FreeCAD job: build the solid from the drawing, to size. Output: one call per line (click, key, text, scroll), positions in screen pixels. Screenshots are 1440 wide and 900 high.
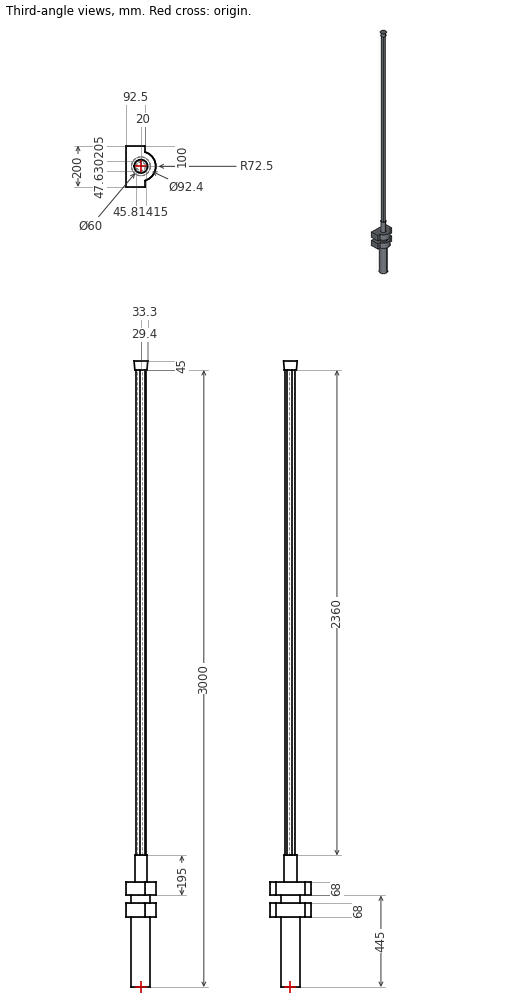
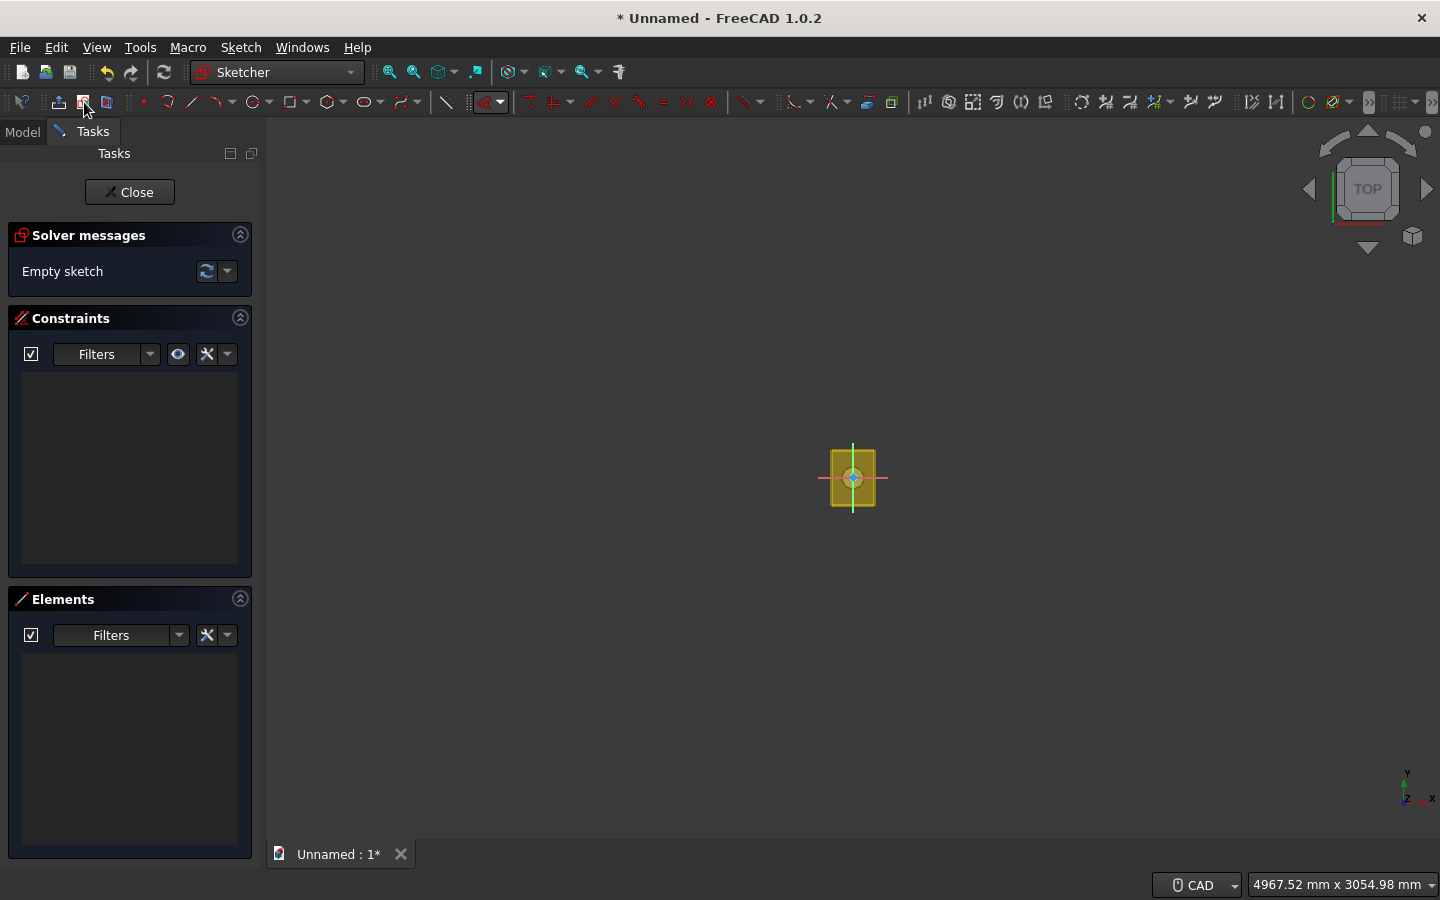
scroll(862, 478, up, 11)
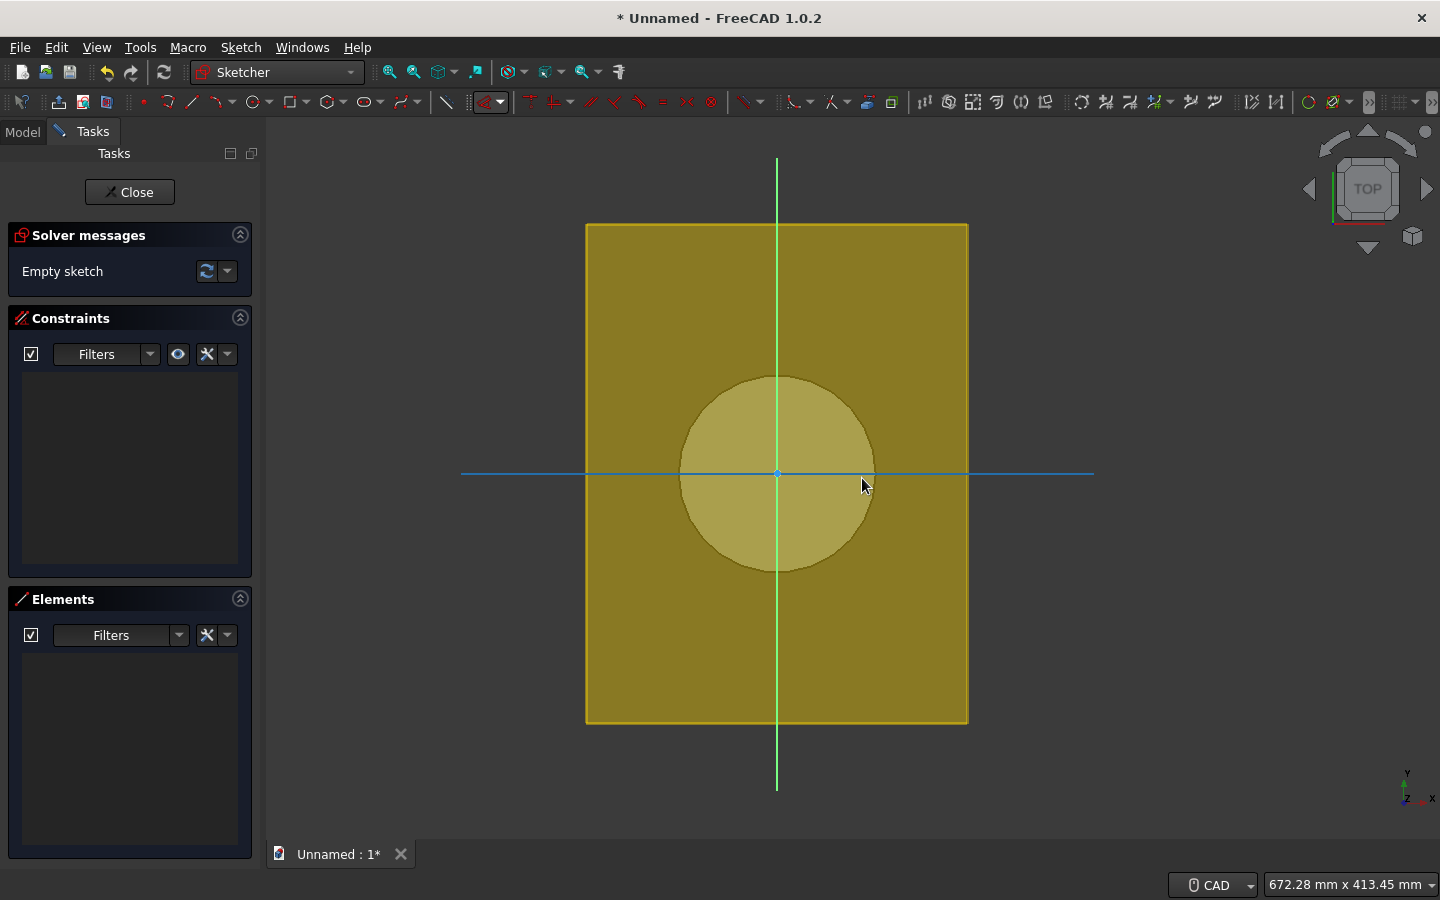
key(g)
key(m)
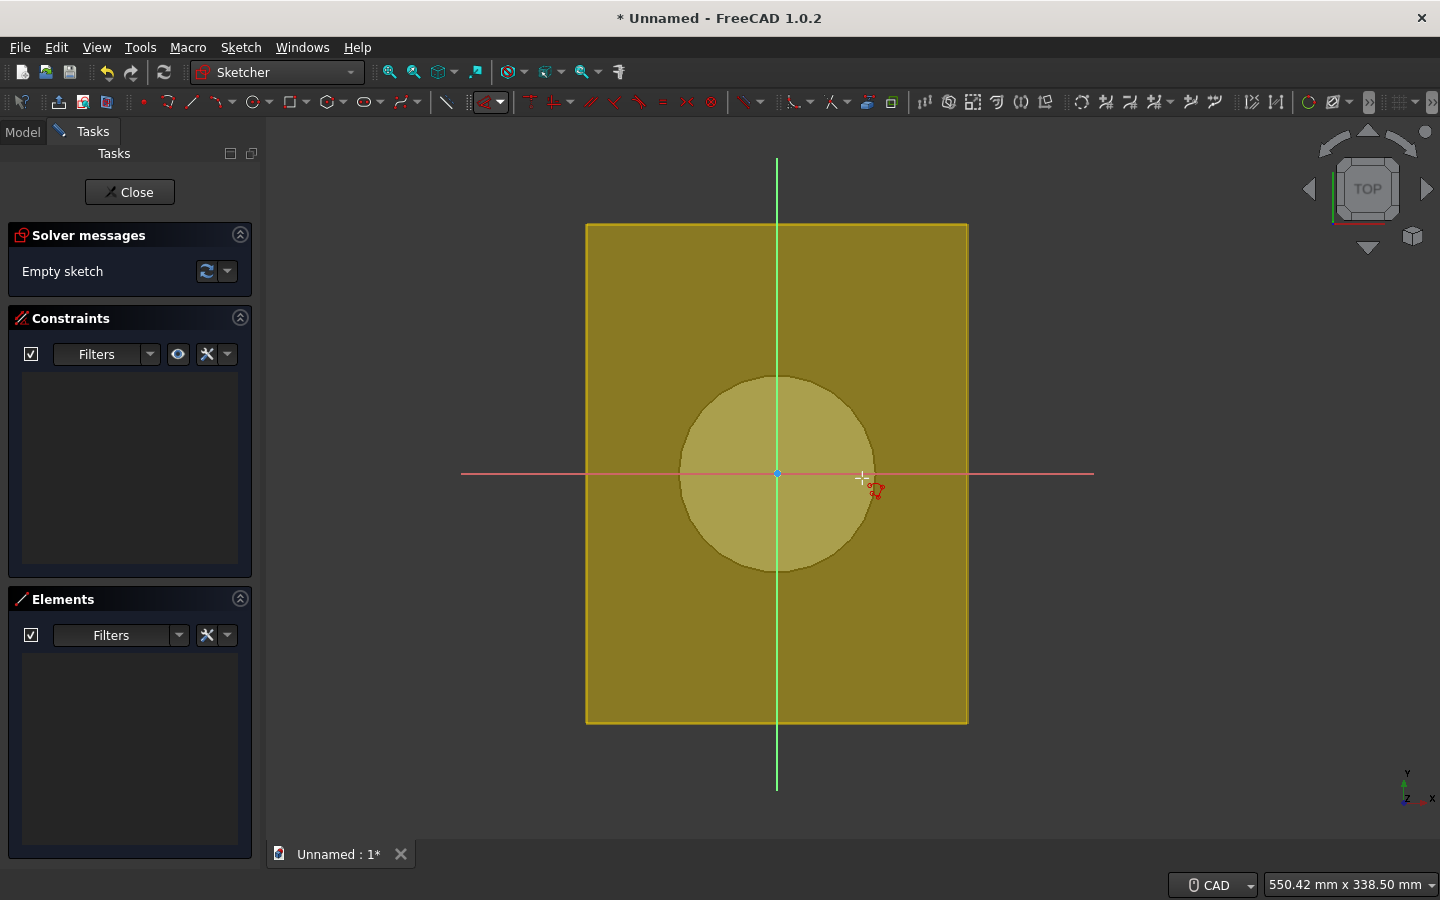
click(820, 325)
click(820, 261)
click(623, 261)
click(623, 687)
click(820, 687)
click(820, 623)
right_click(820, 623)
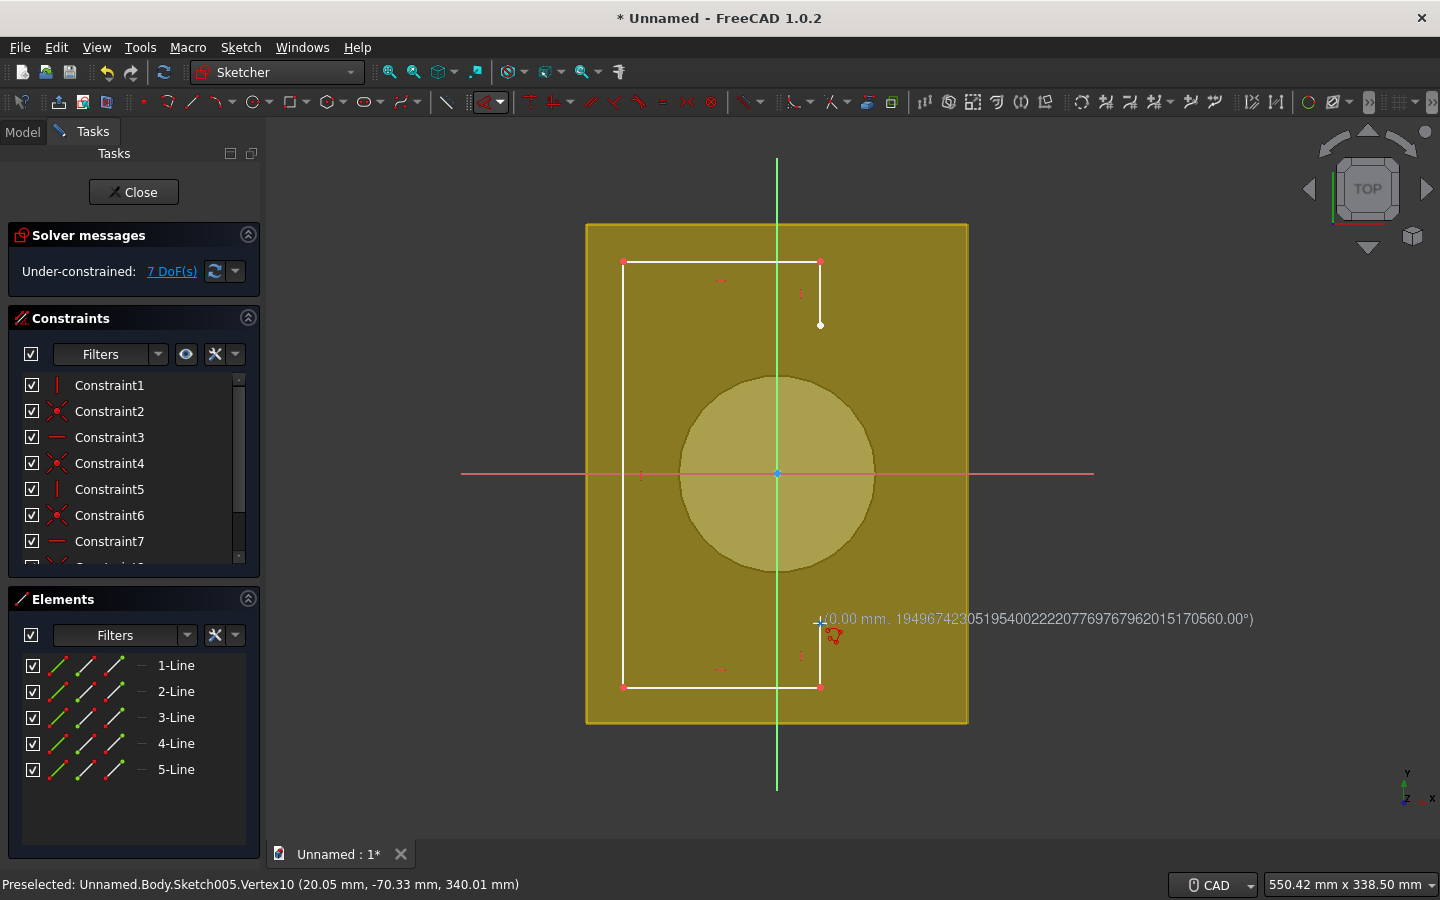
key(g)
key(3)
key(a)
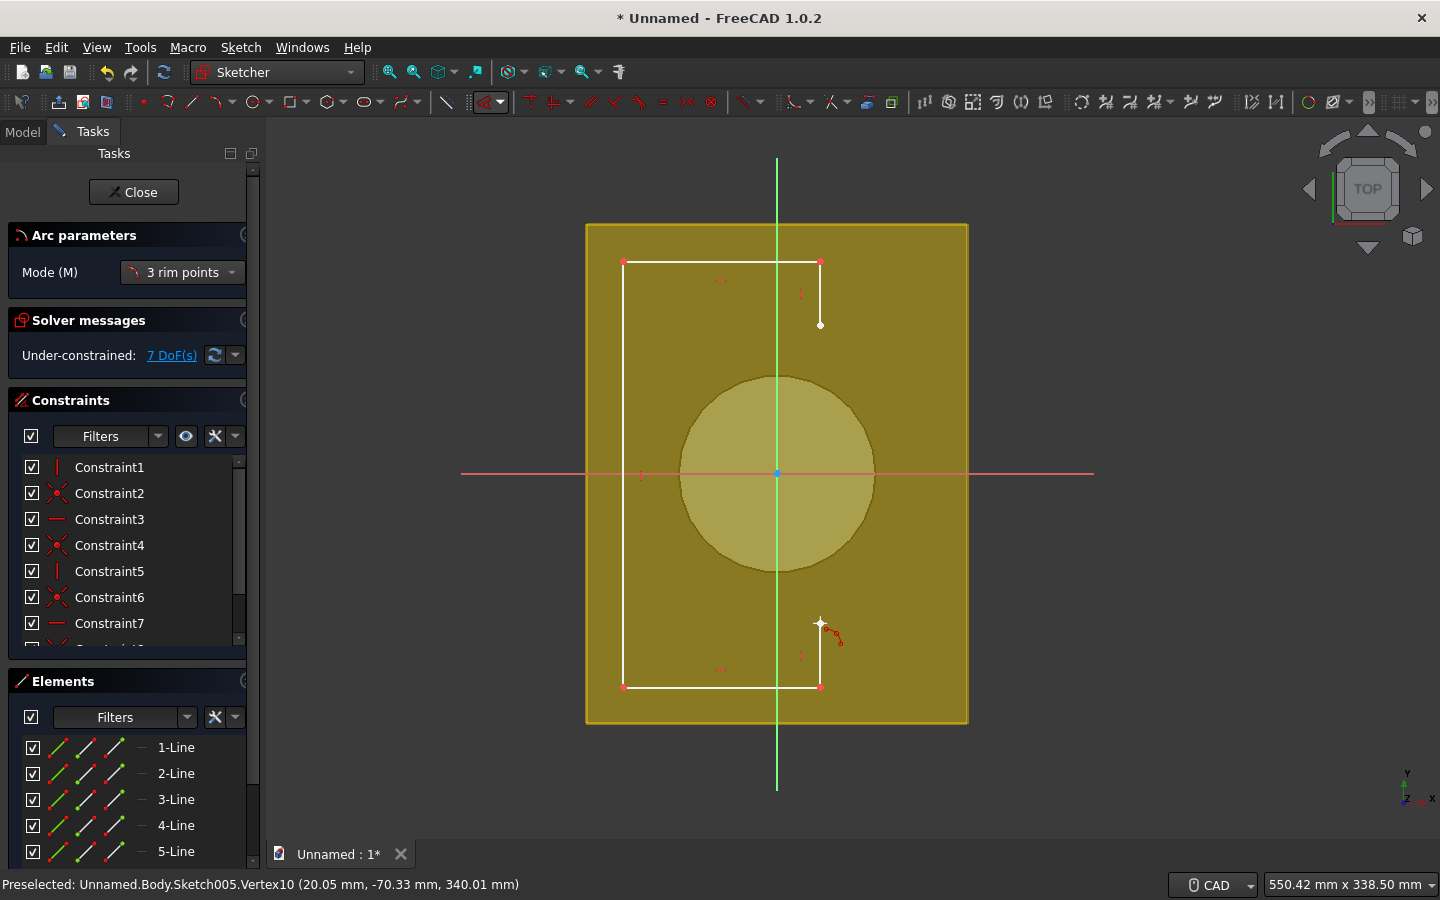
click(820, 624)
click(820, 326)
click(927, 513)
key(Escape)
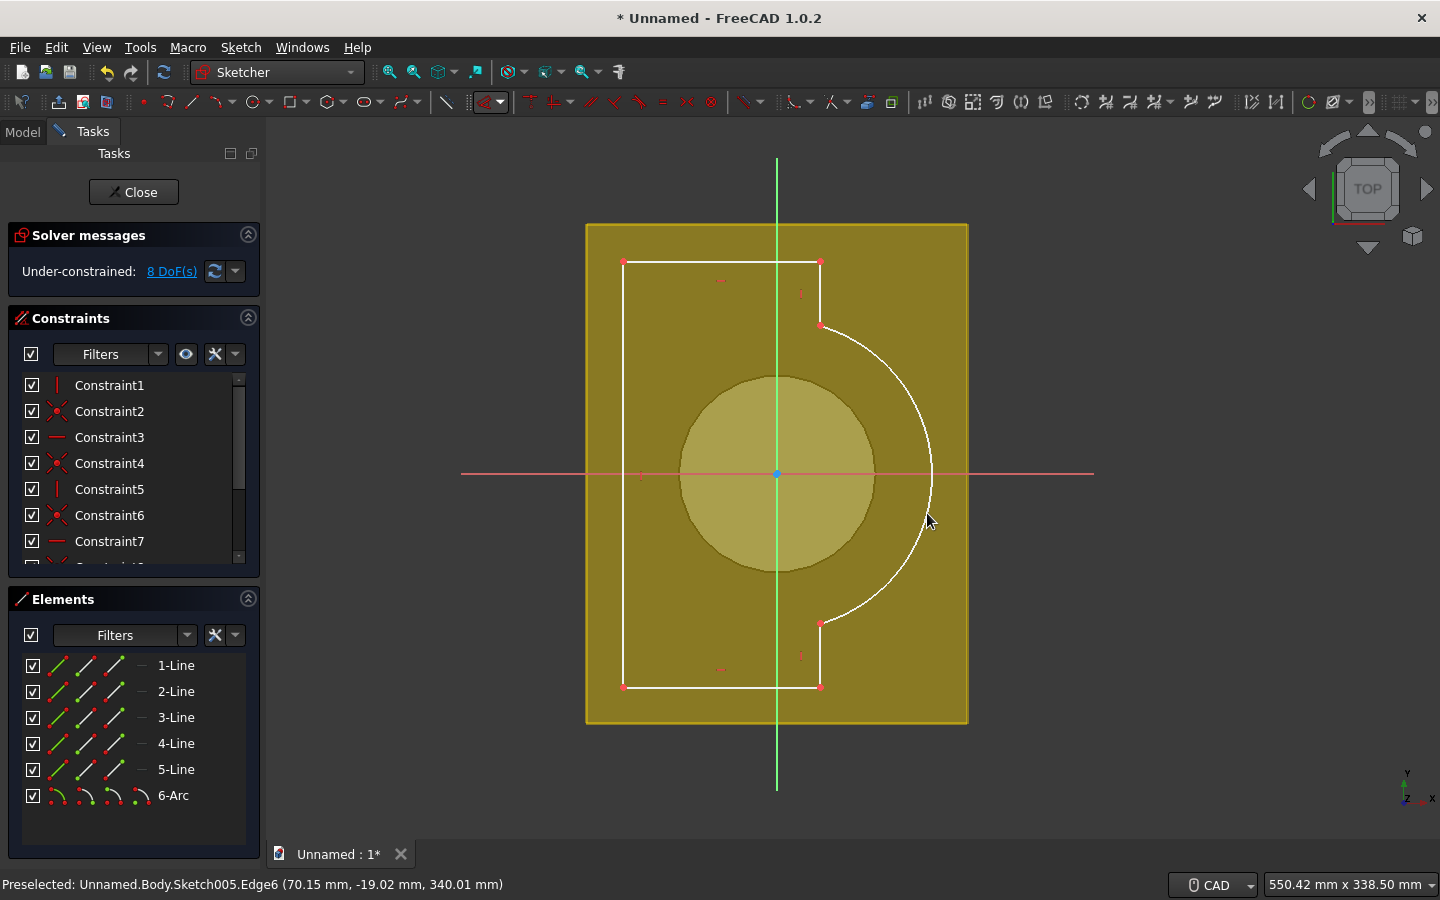
drag(767, 464, 787, 485)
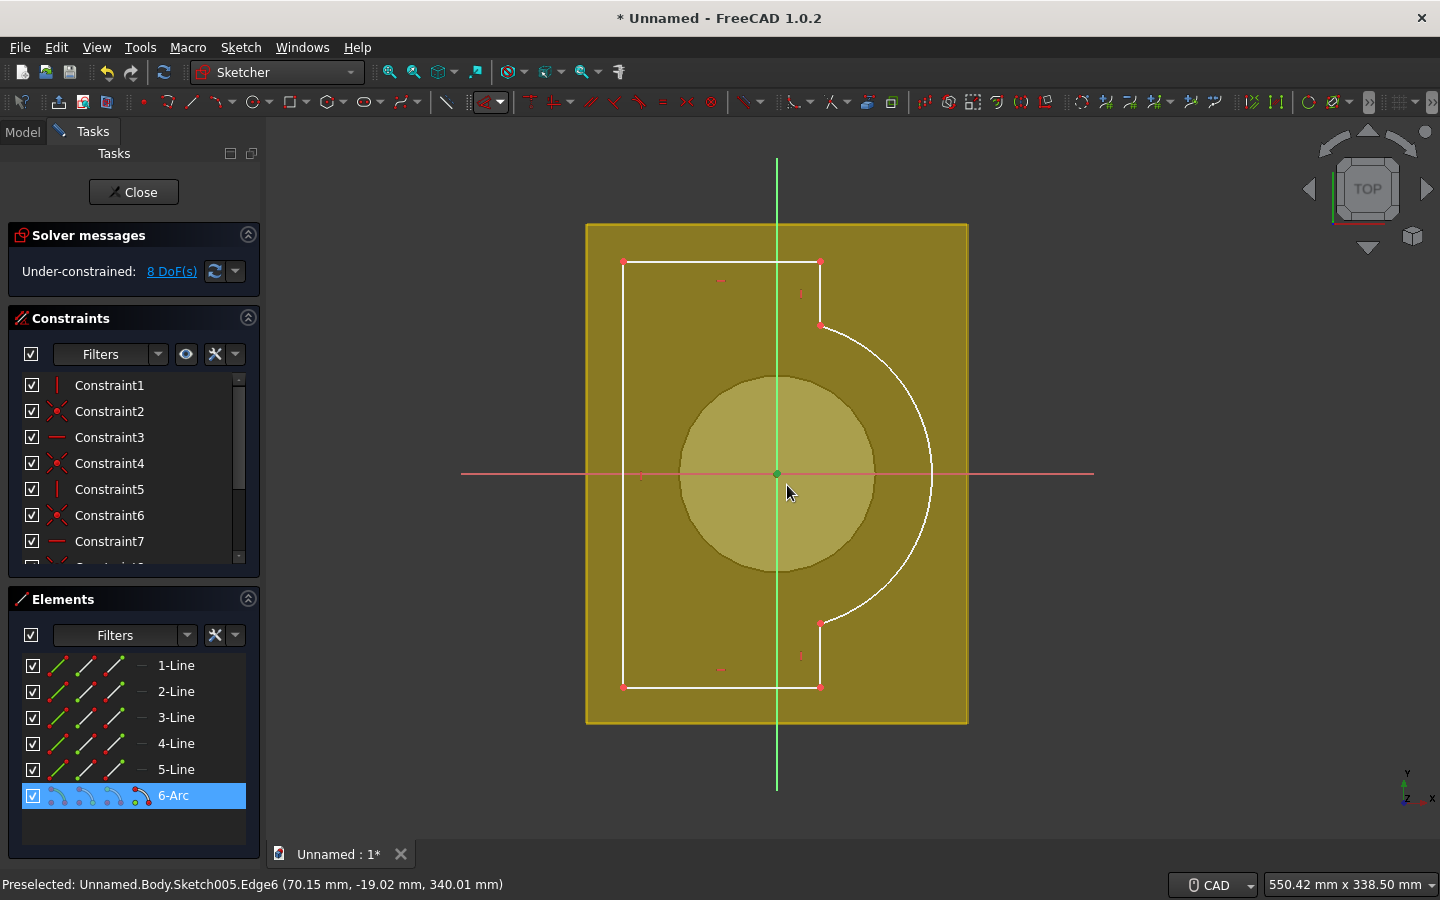
key(c)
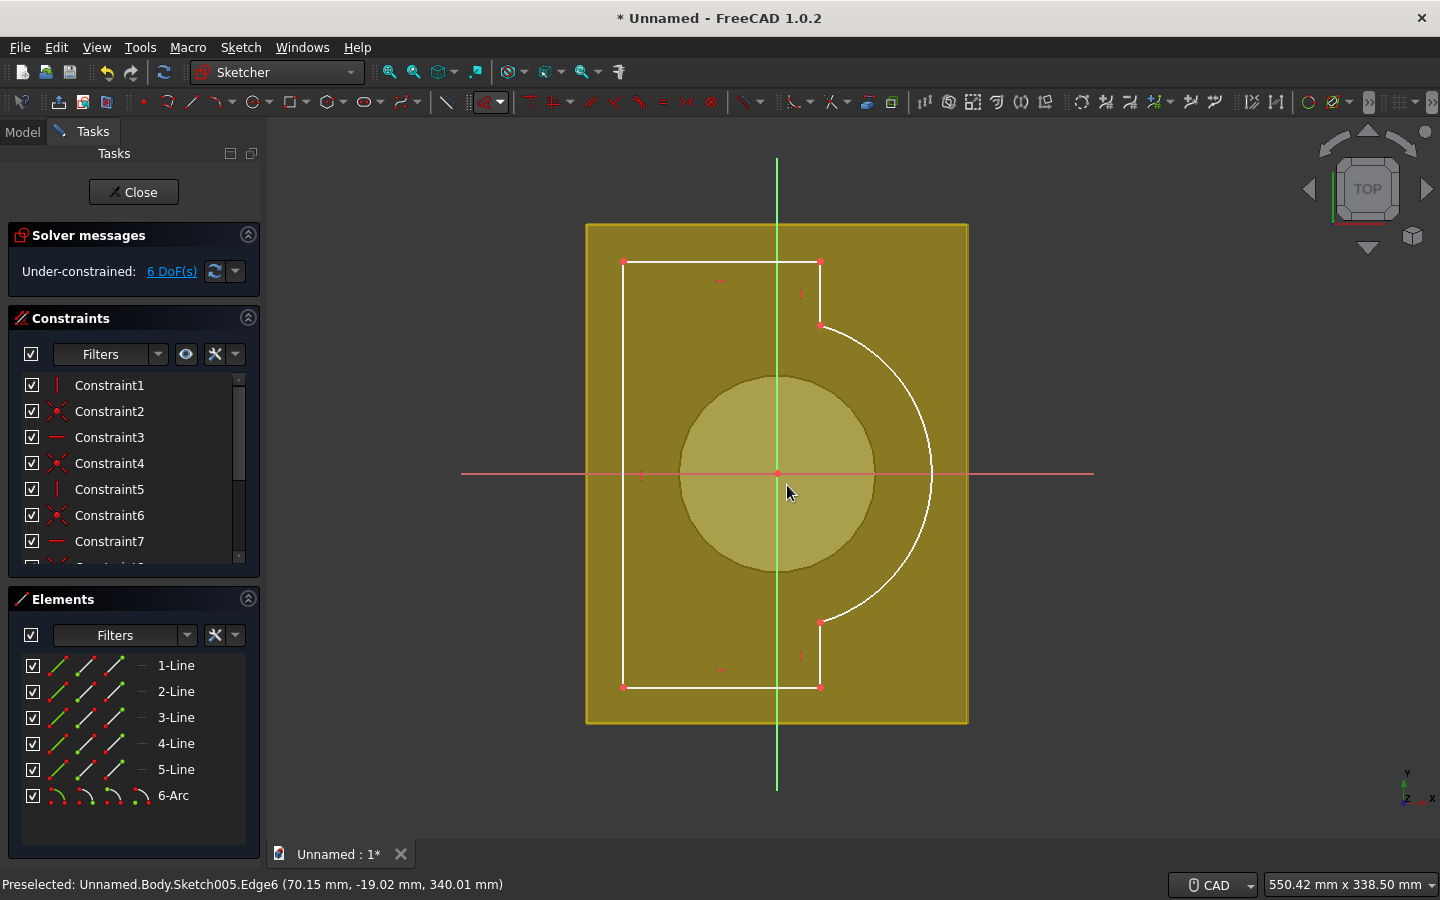
click(912, 550)